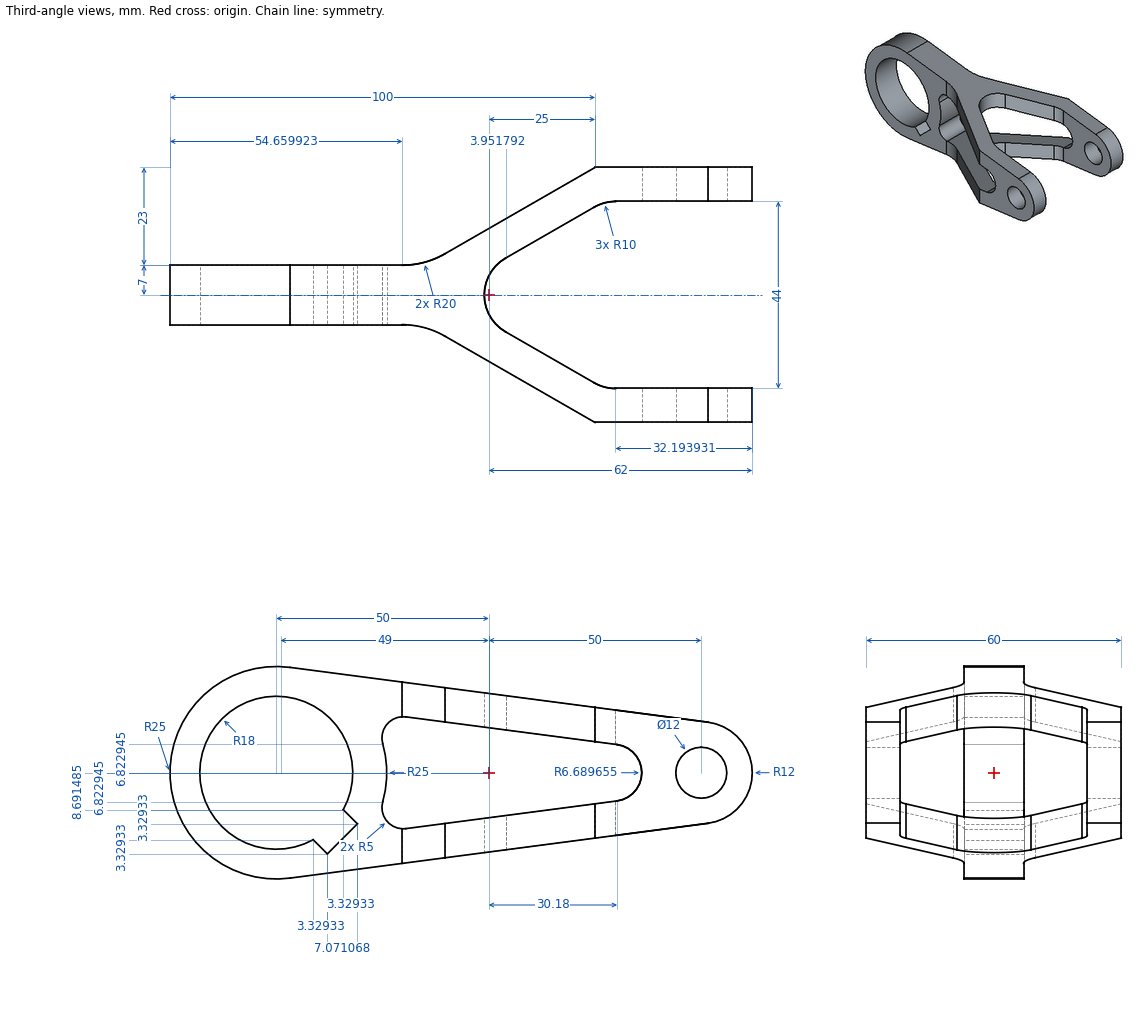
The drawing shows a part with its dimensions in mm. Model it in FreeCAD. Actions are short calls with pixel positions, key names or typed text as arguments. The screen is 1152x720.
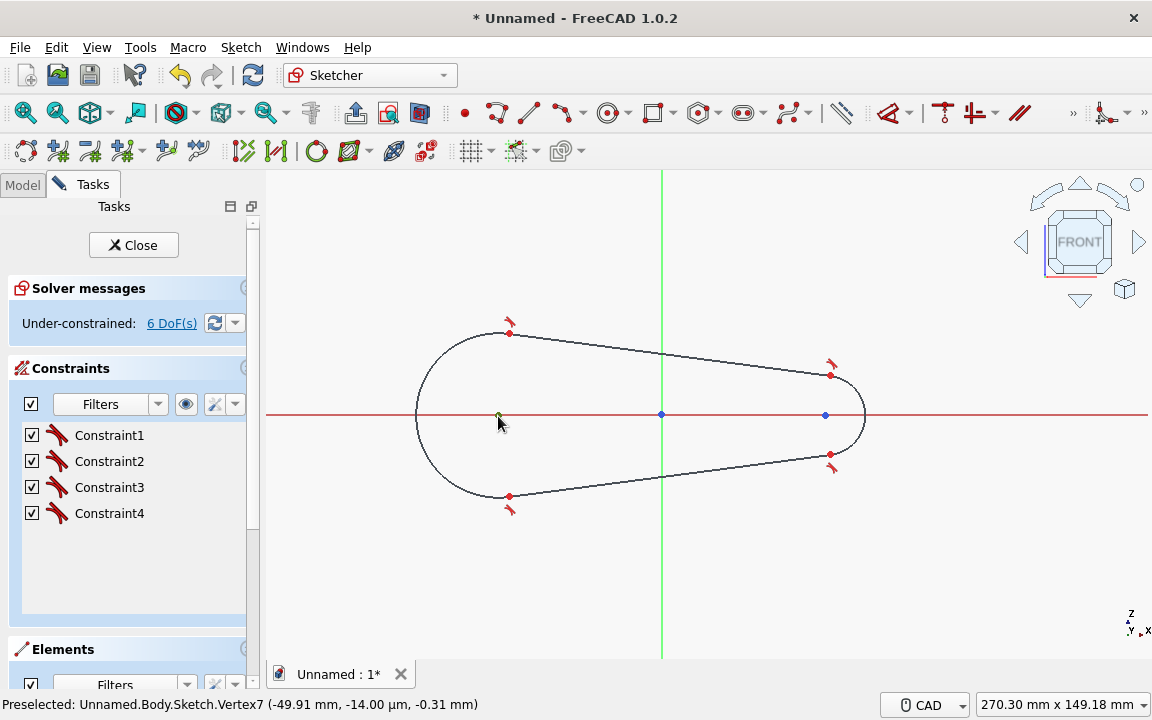
click(344, 414)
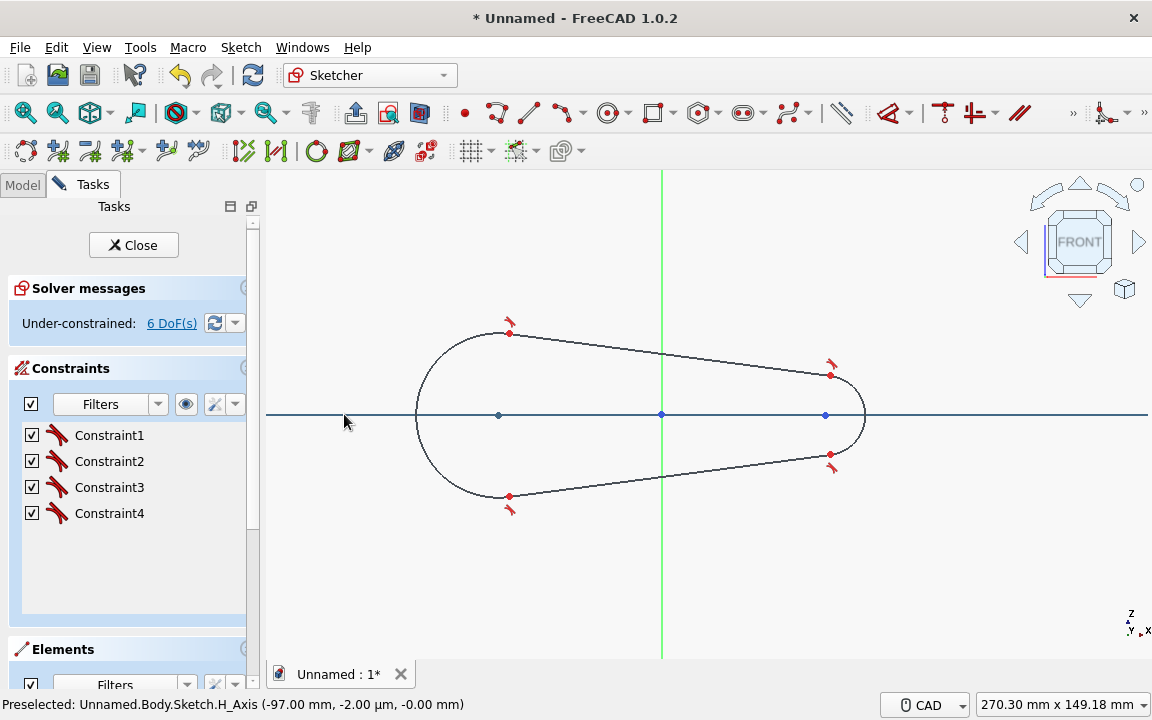
key(c)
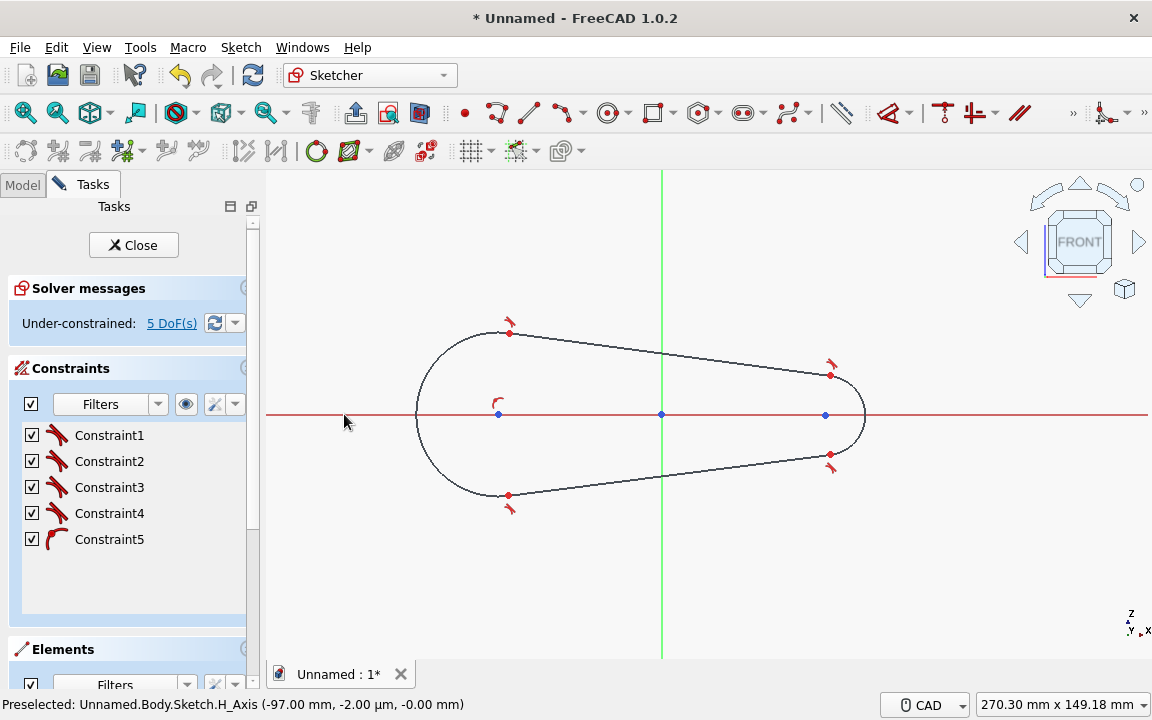
click(825, 415)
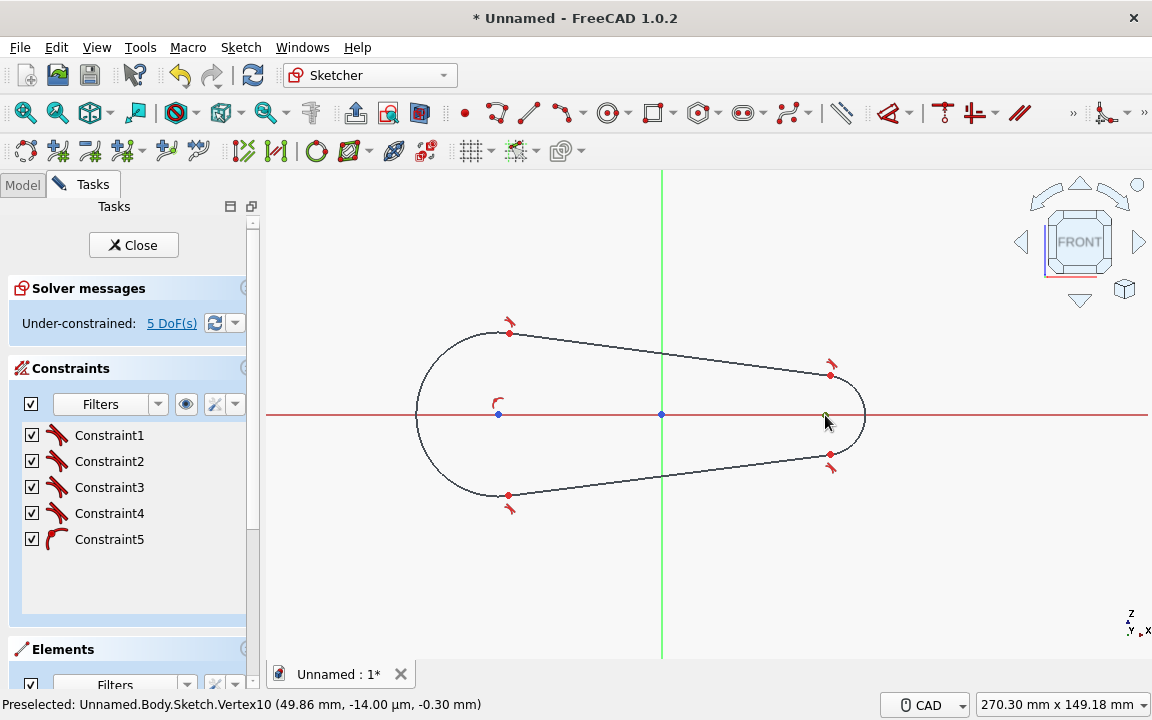
click(344, 414)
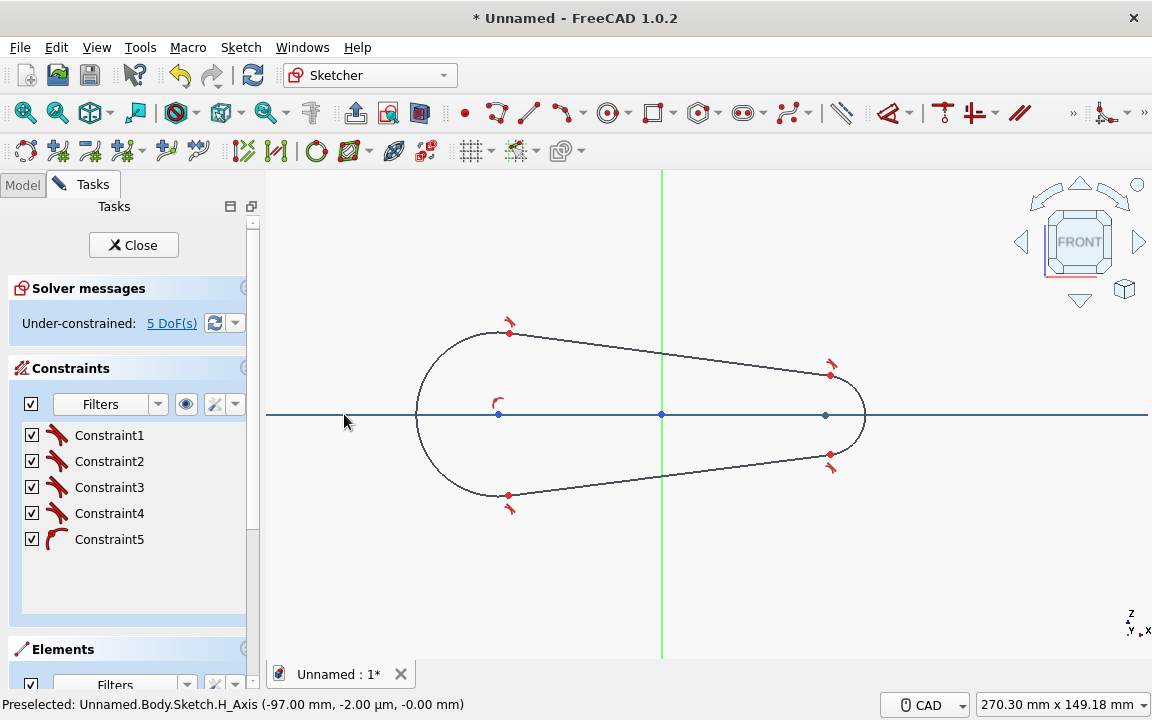
click(944, 114)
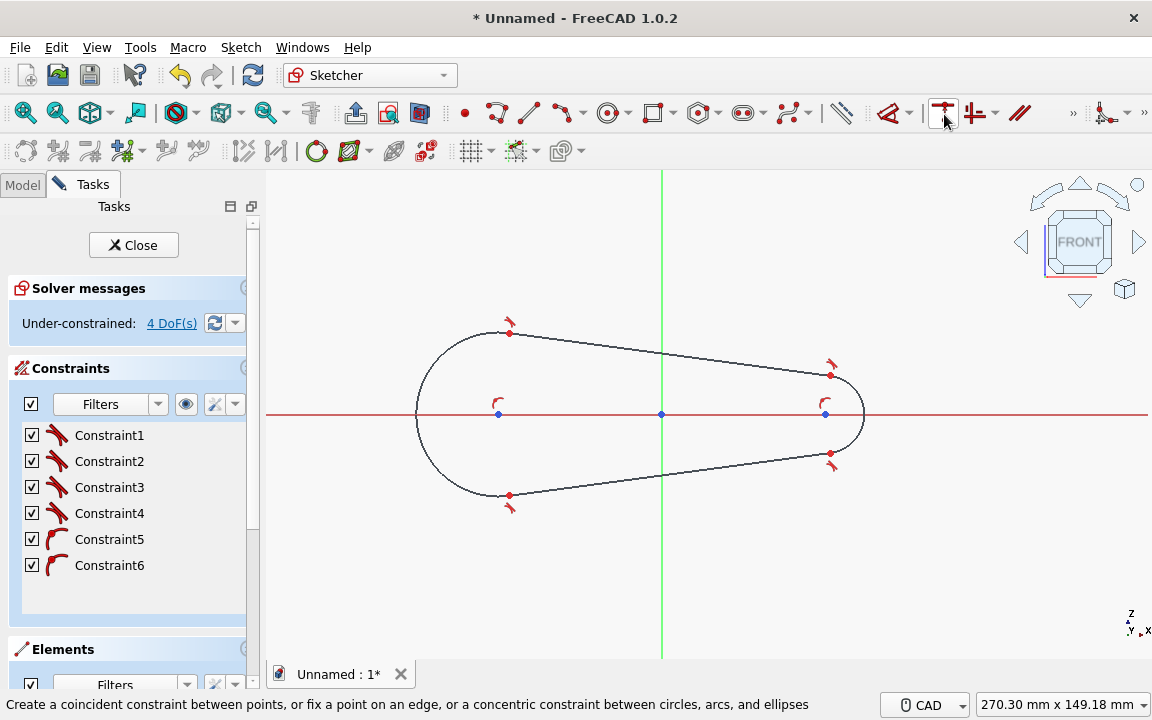
click(888, 114)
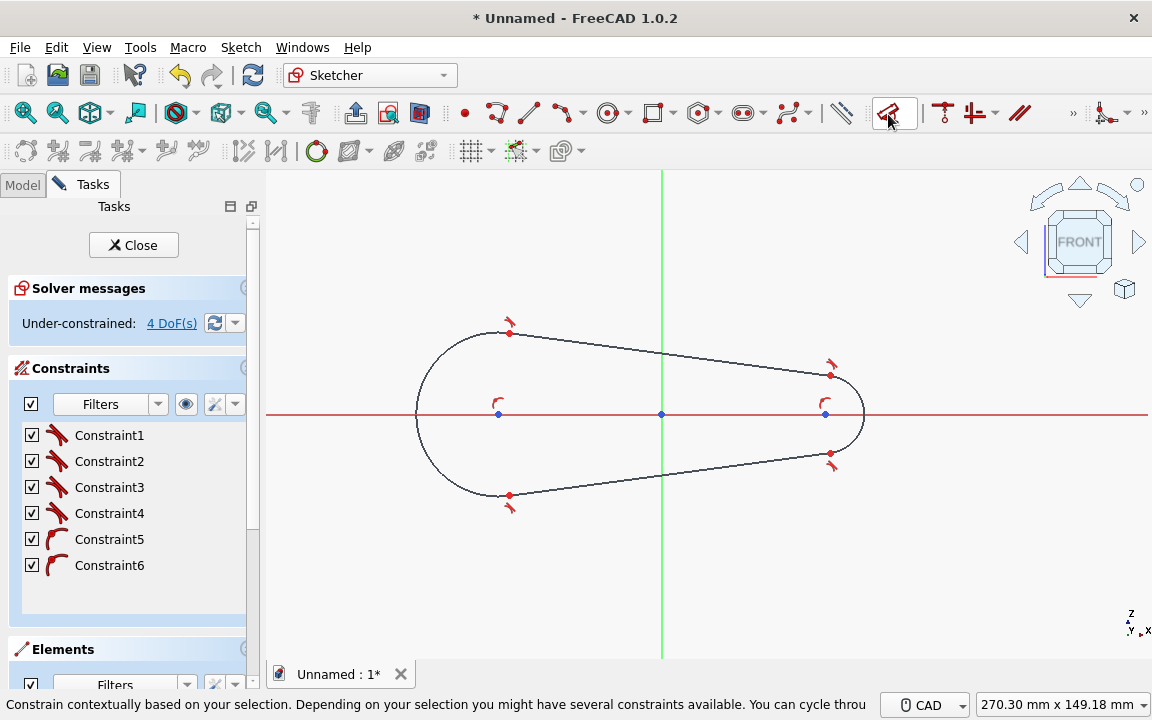
click(435, 363)
click(410, 343)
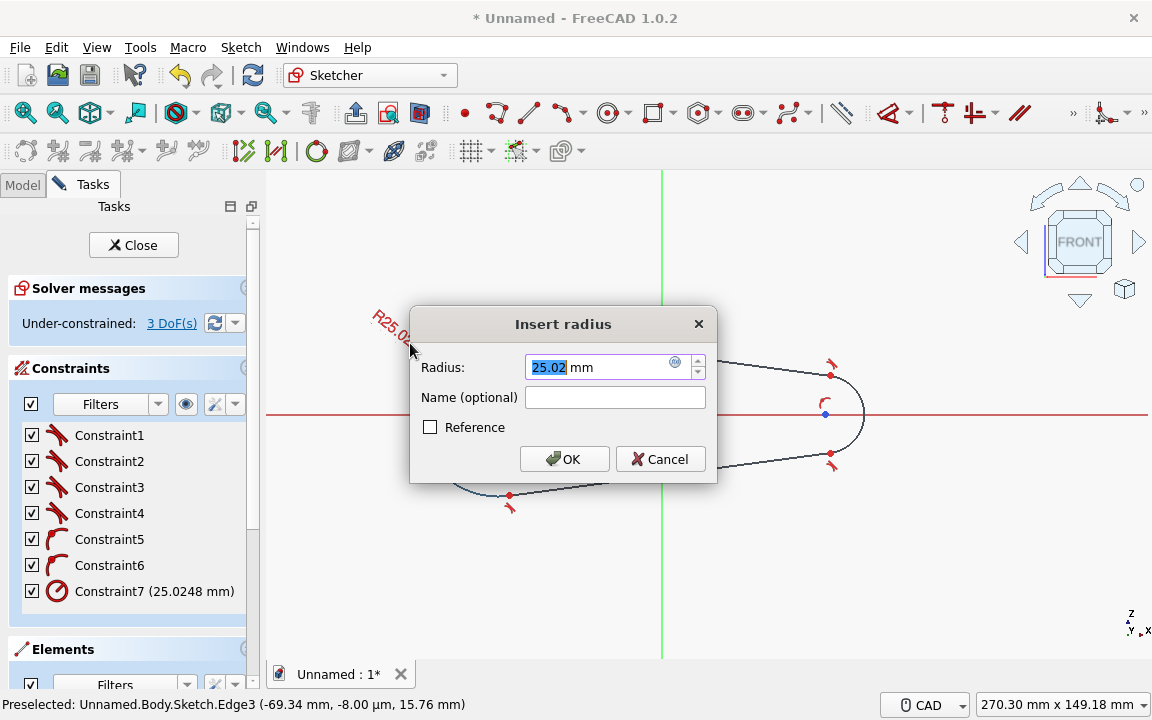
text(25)
key(Return)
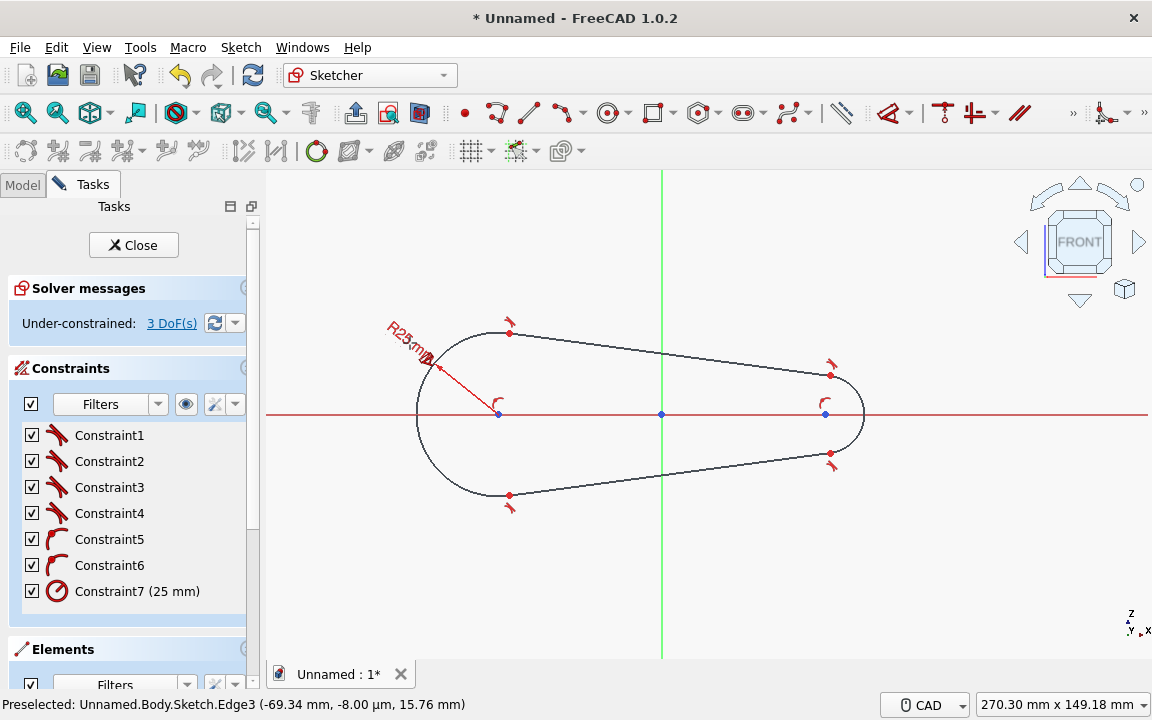
click(858, 436)
click(885, 454)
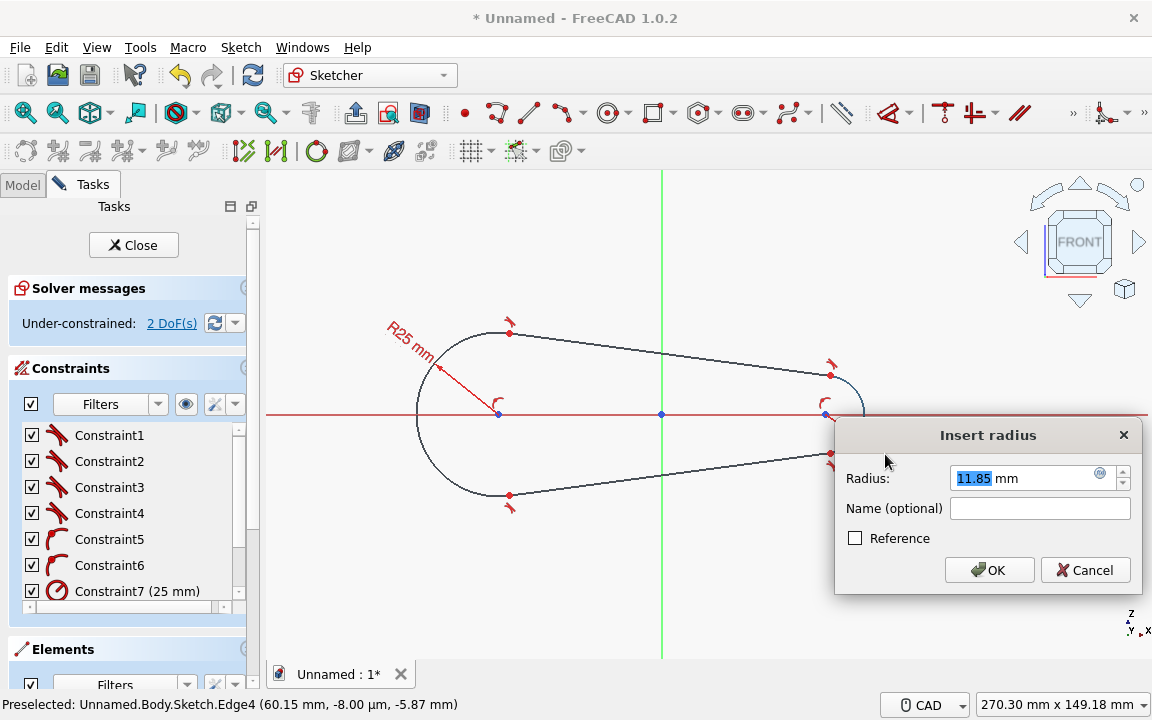
text(12)
key(Return)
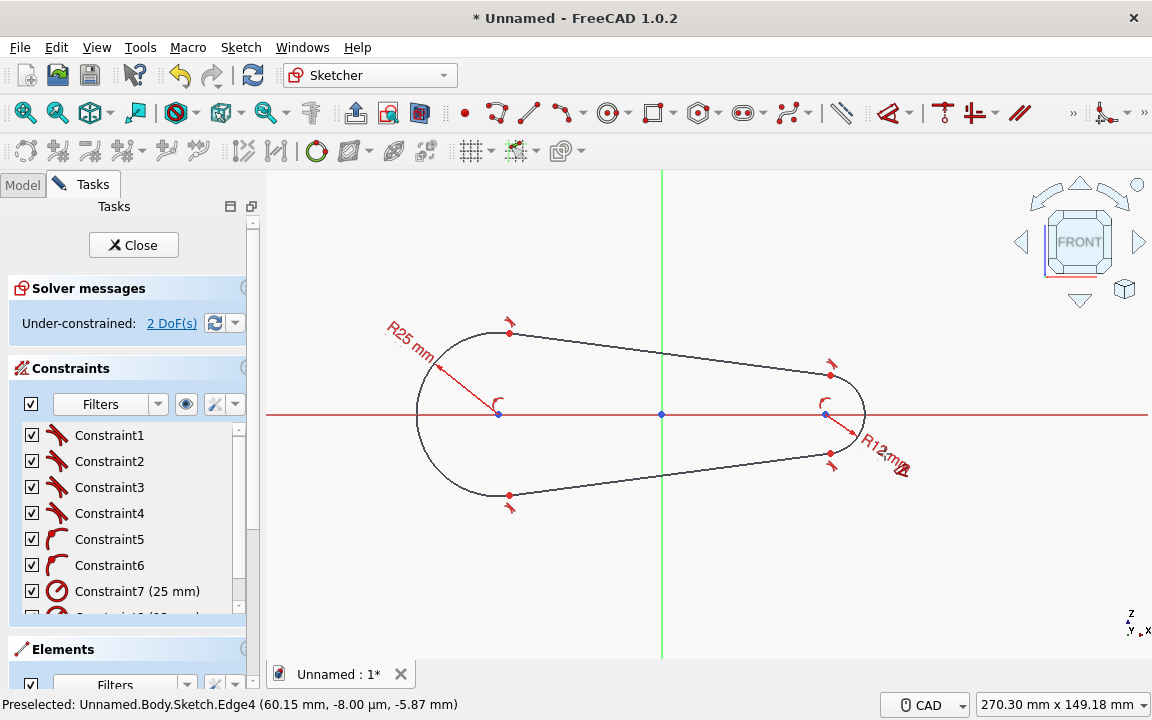
click(499, 414)
click(580, 448)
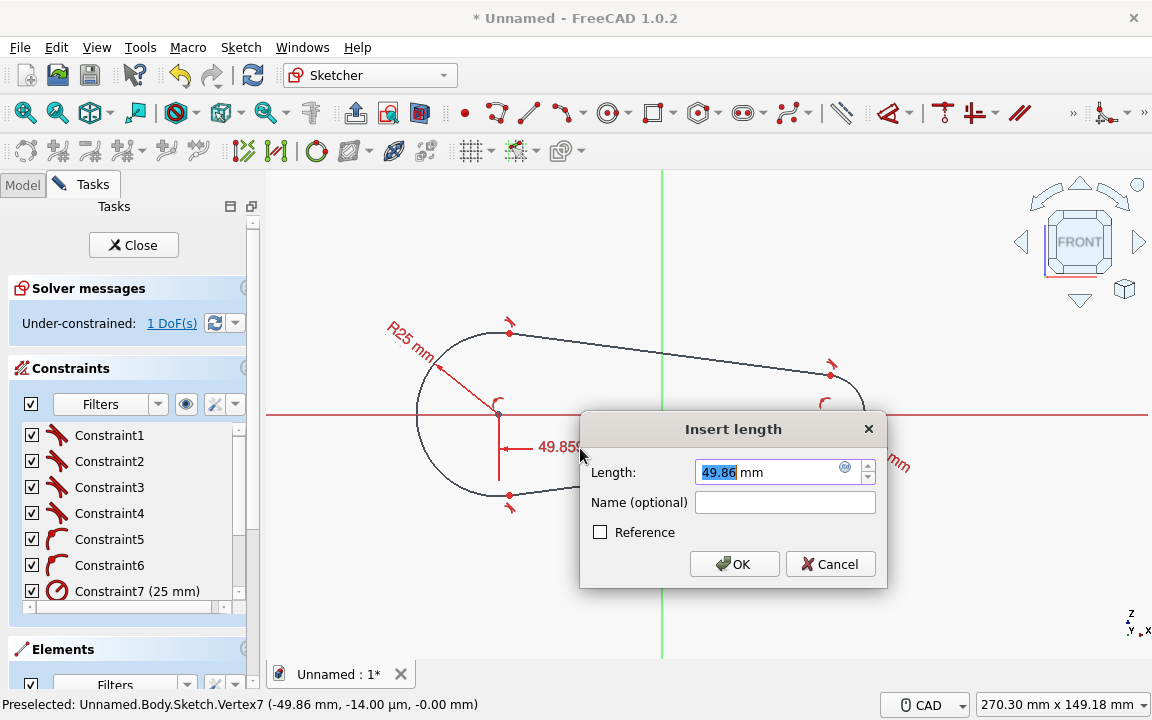
text(50)
key(Return)